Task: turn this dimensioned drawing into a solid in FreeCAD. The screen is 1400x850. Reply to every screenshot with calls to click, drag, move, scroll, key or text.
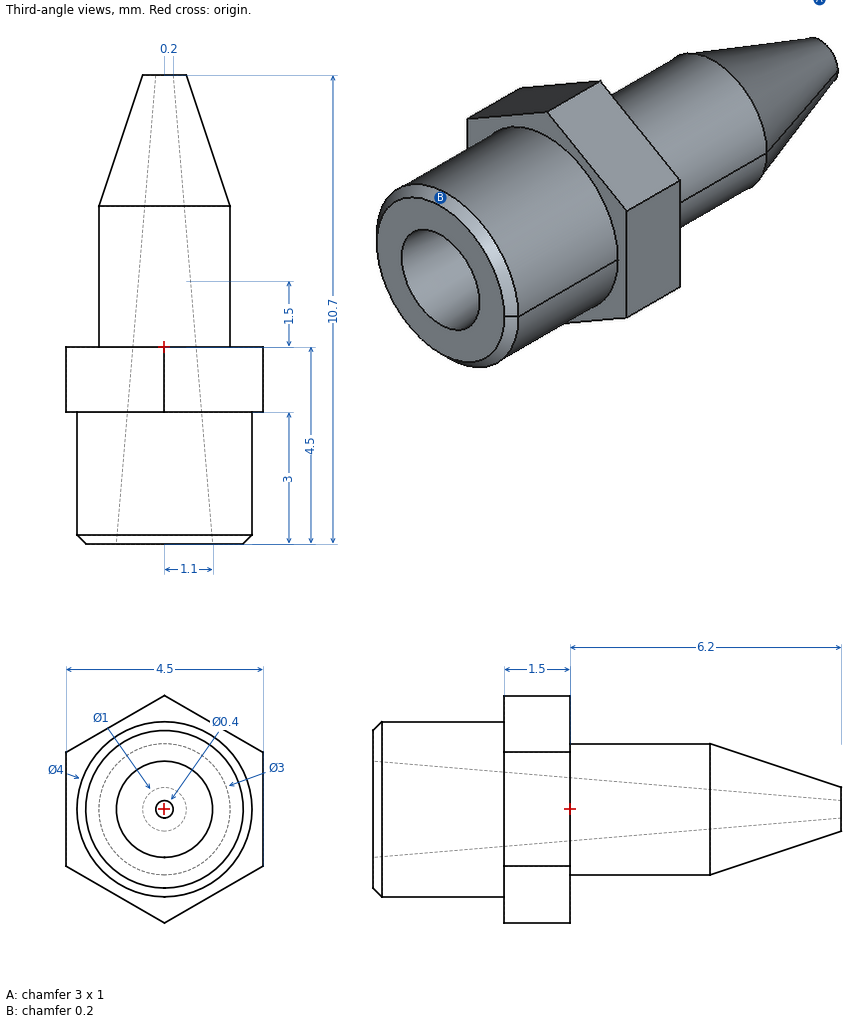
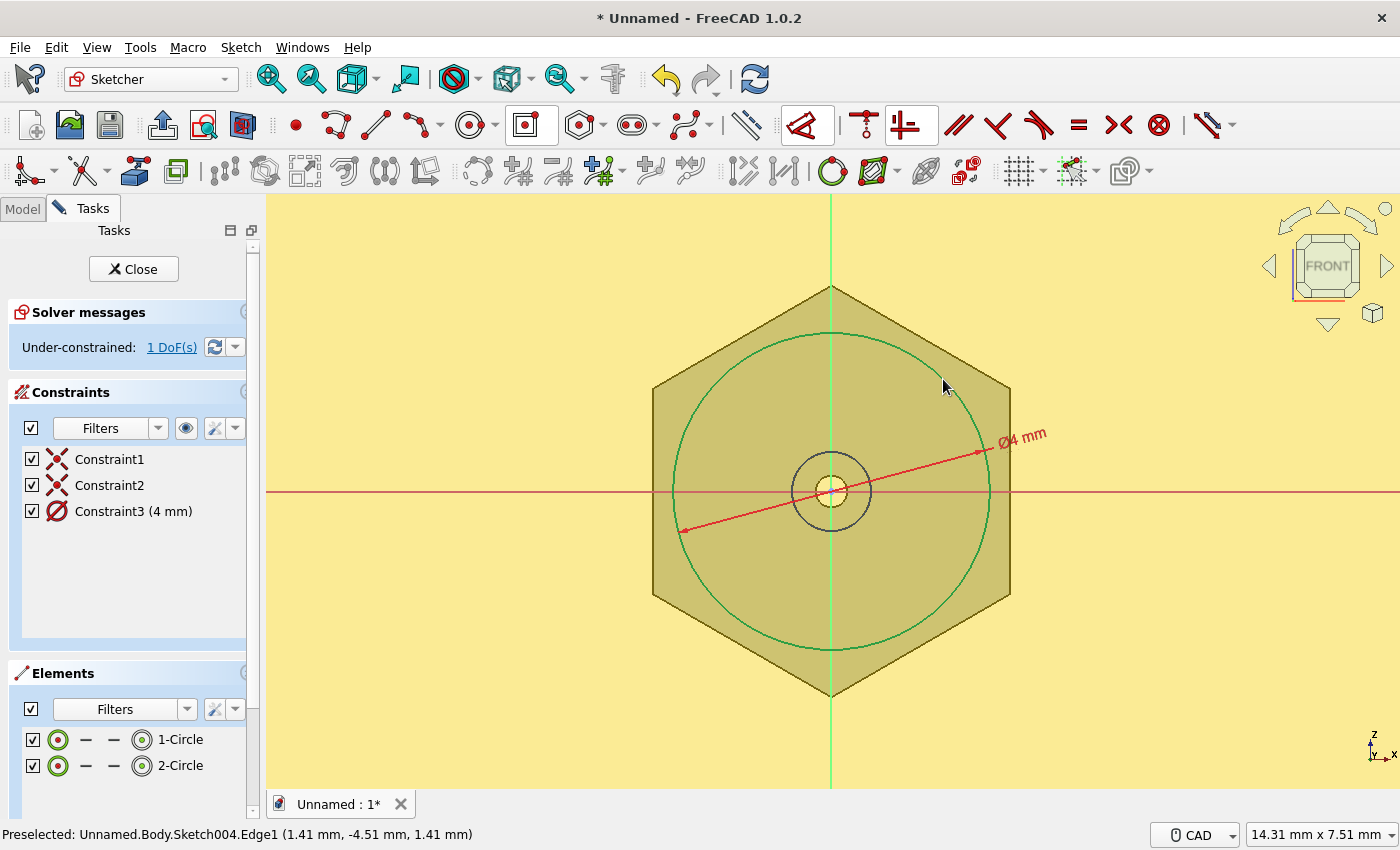
click(859, 463)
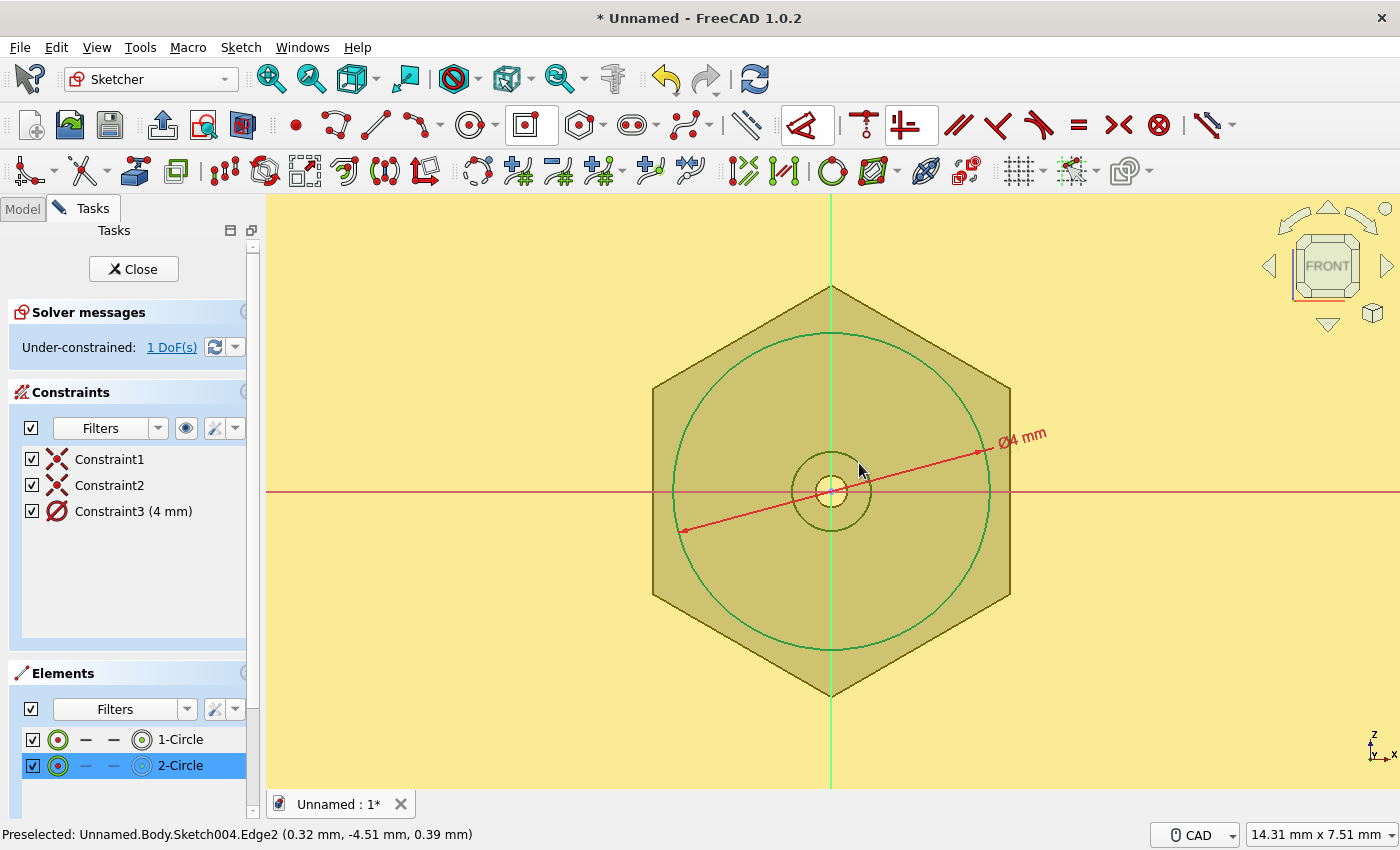
click(828, 126)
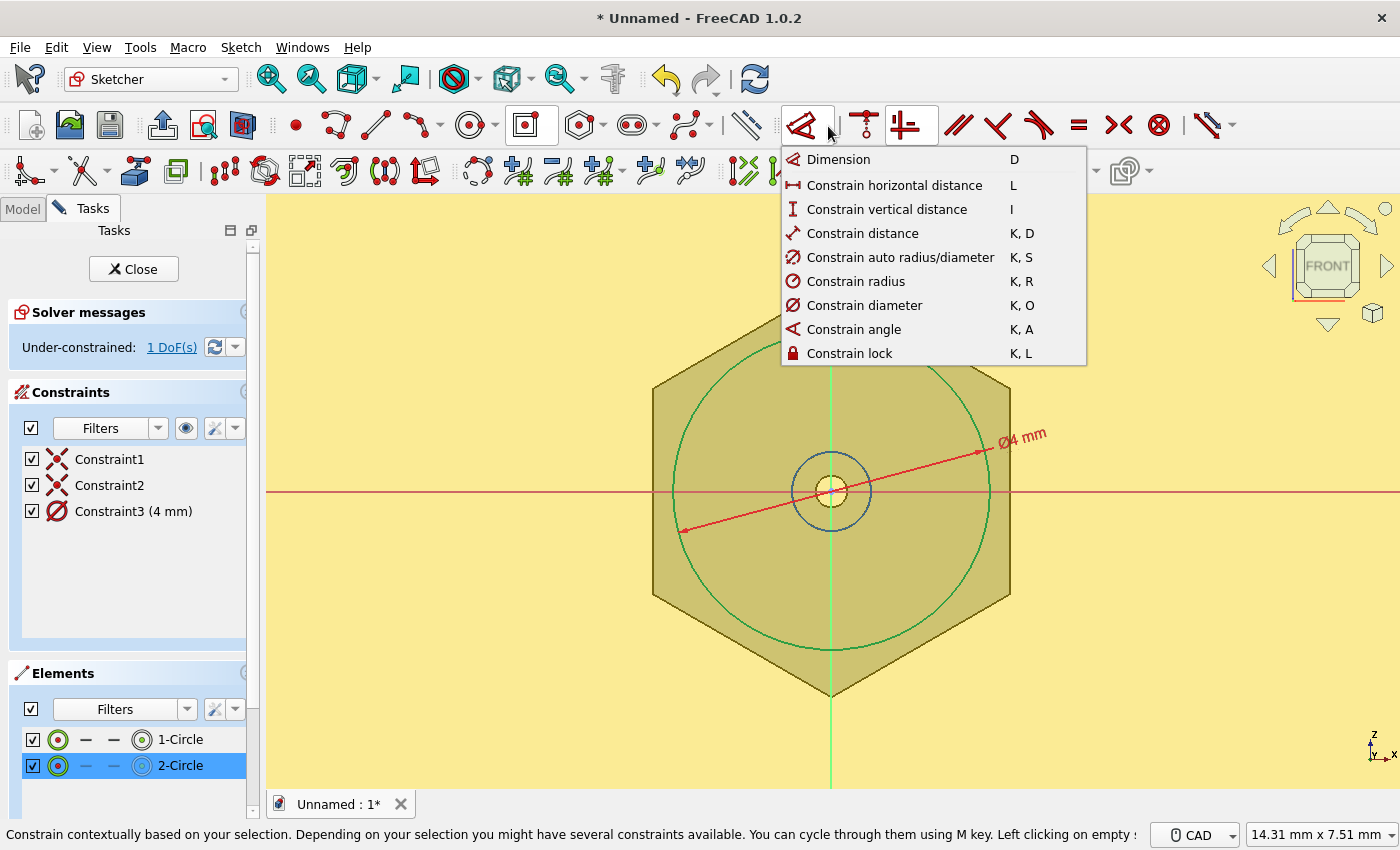
click(934, 305)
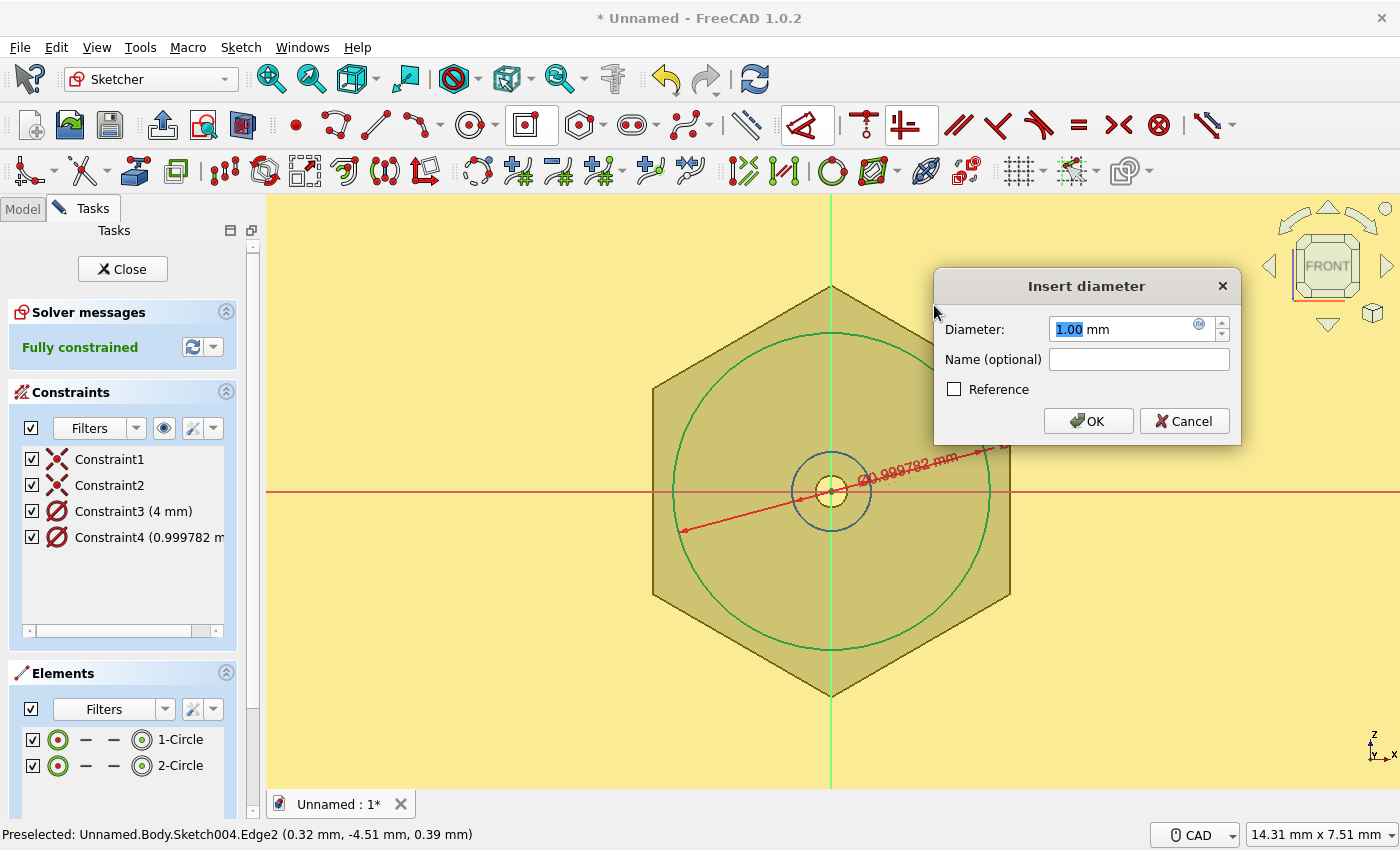
text(1)
key(Return)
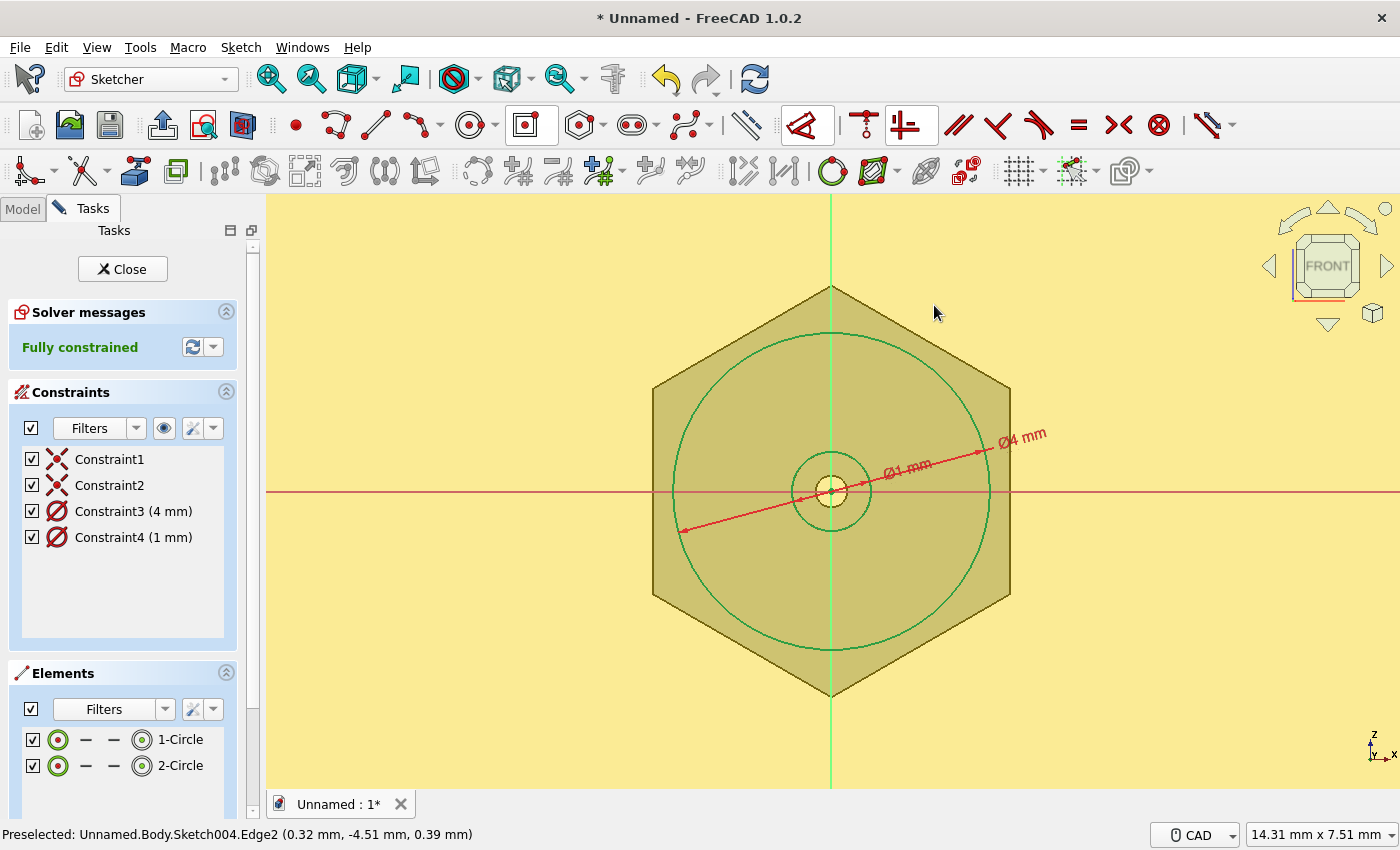
click(123, 269)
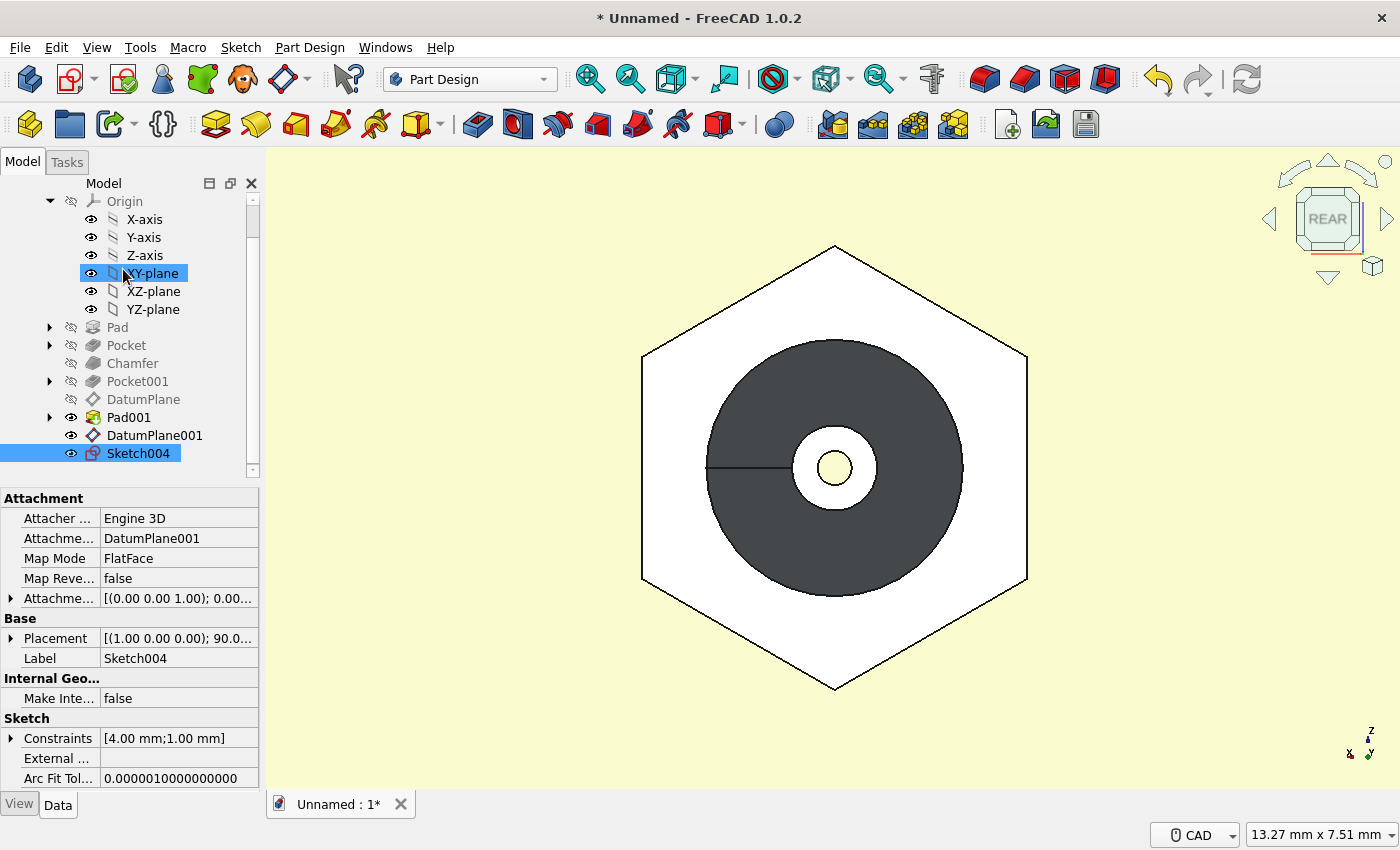
click(216, 124)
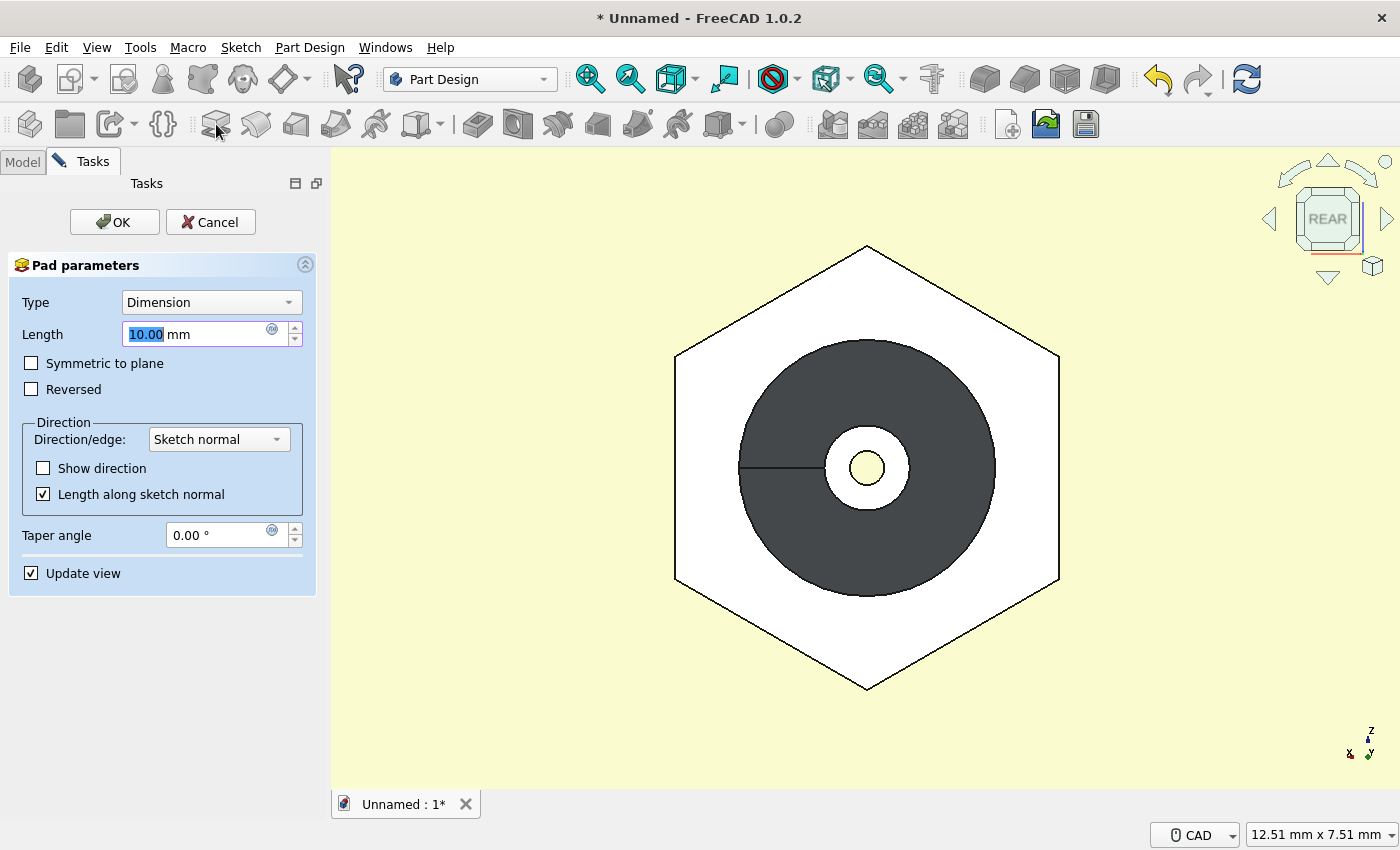
text(3)
key(Tab)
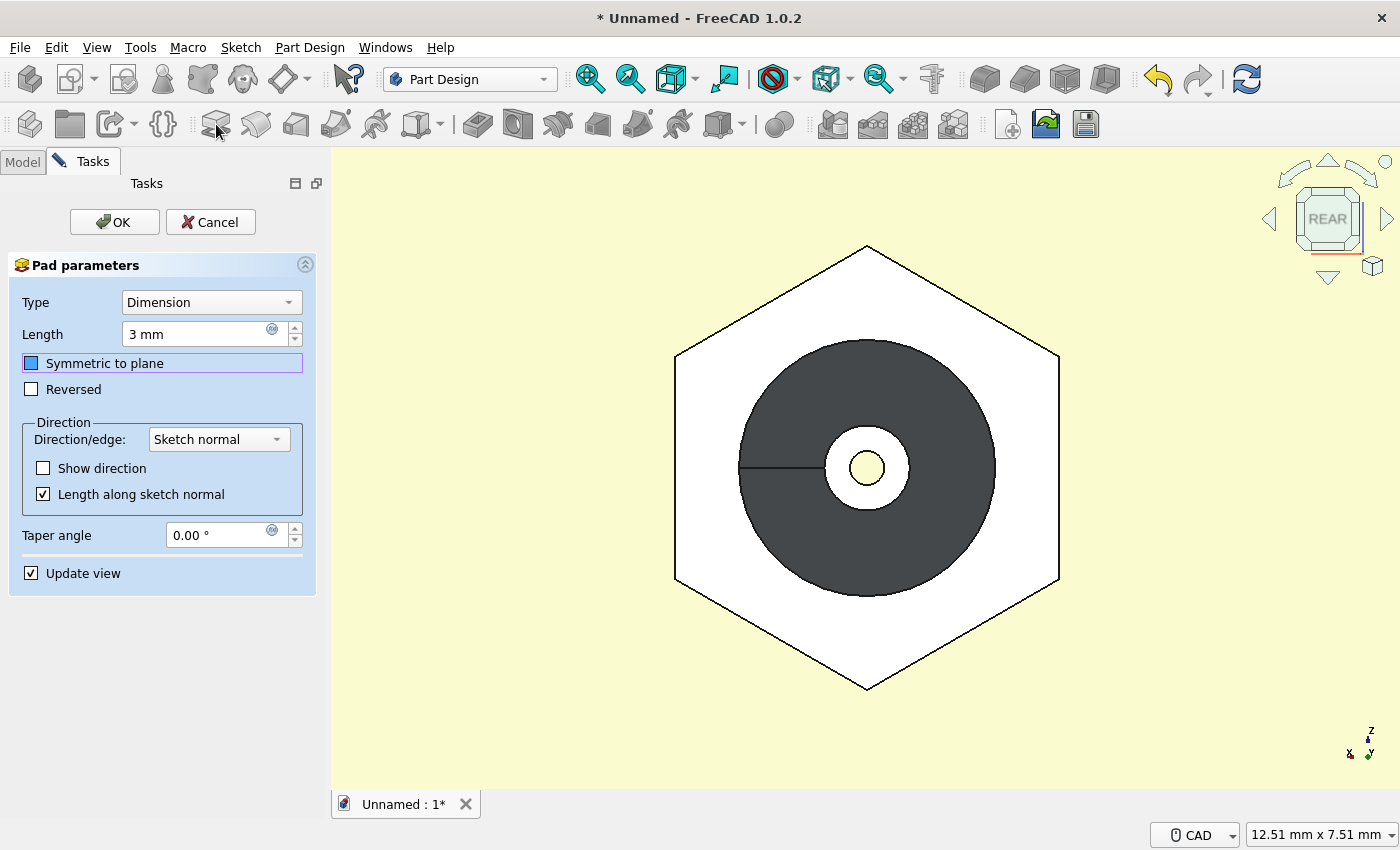
click(30, 389)